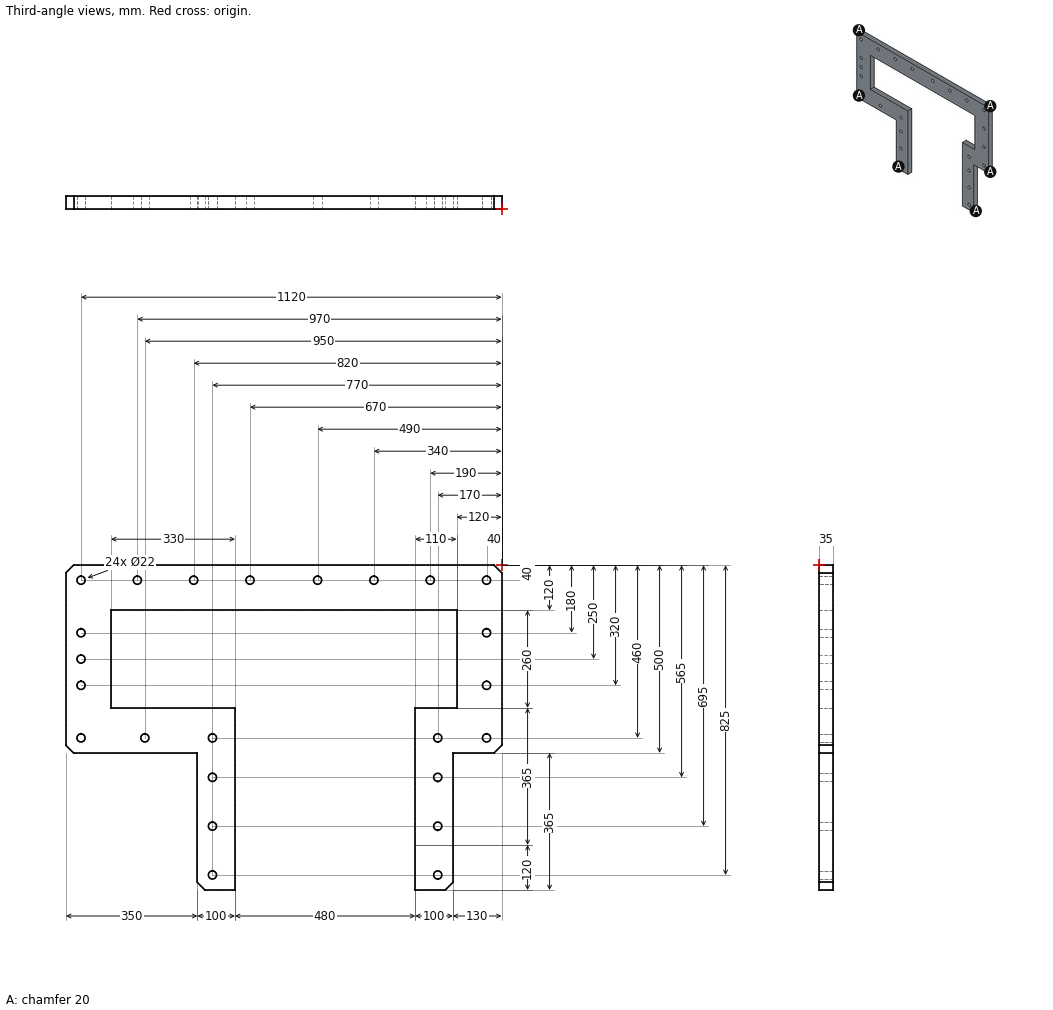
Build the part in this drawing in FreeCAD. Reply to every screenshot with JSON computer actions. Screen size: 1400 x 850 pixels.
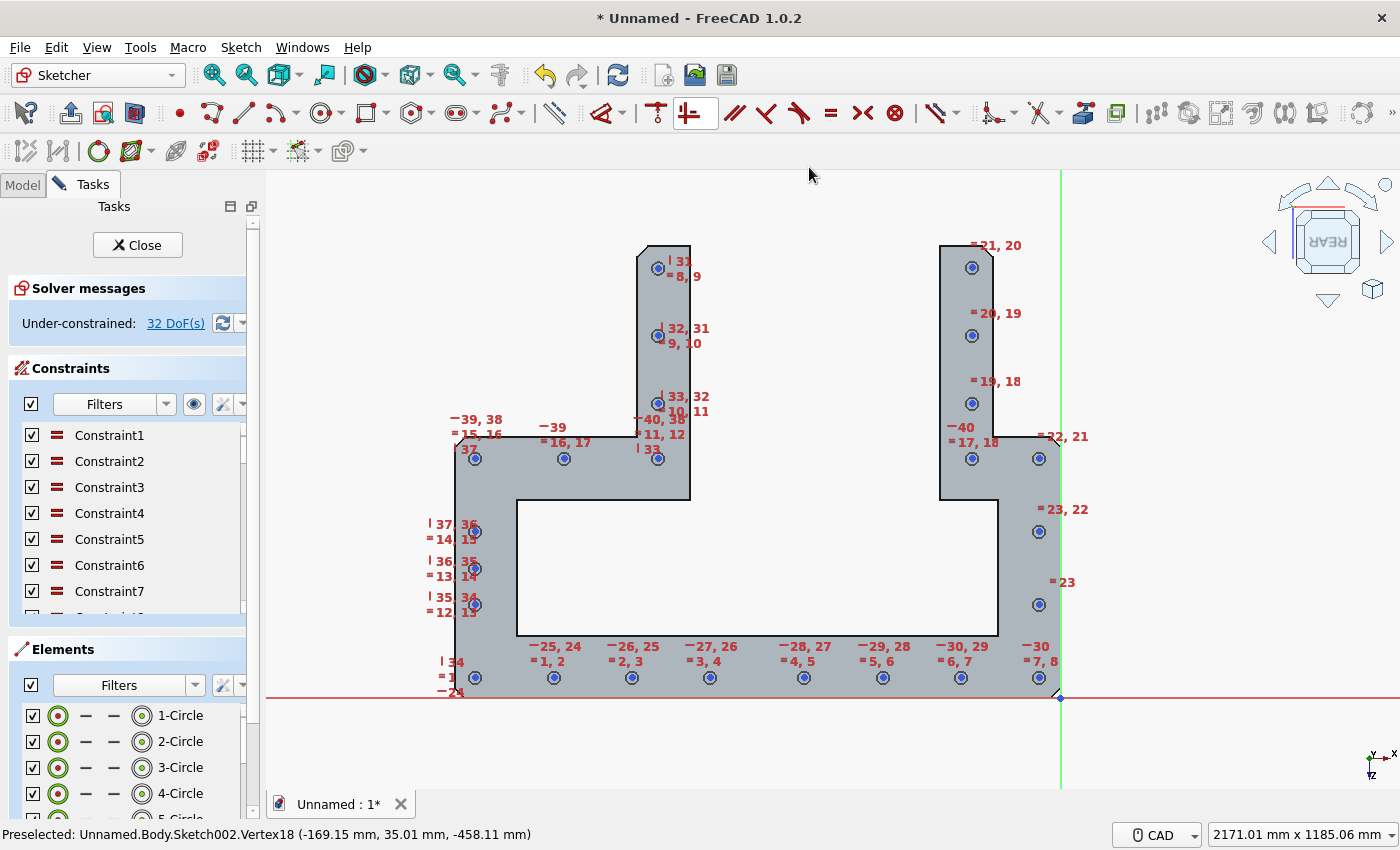
{"action": "left_click", "coordinate": [972, 459]}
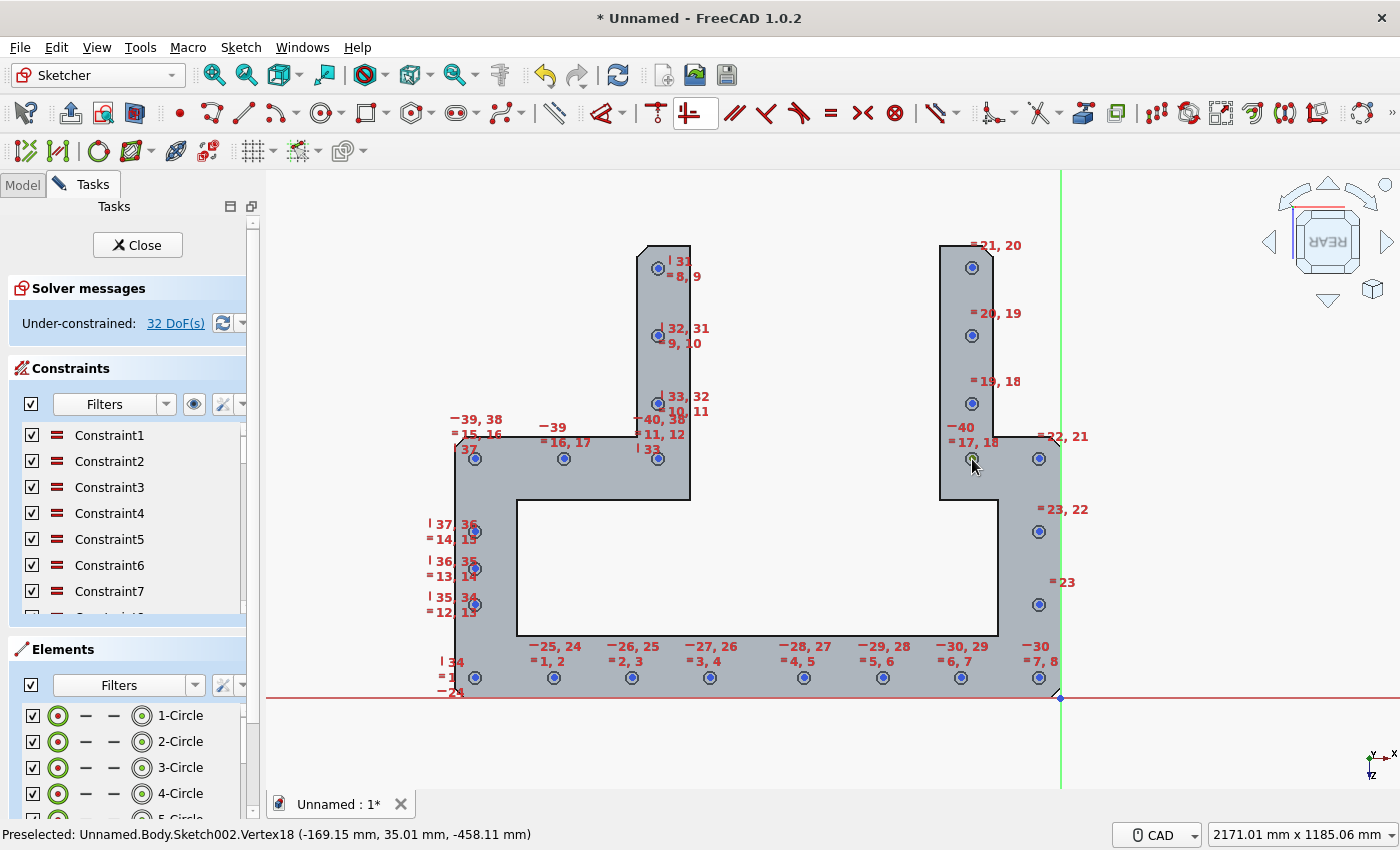
{"action": "left_click", "coordinate": [972, 404]}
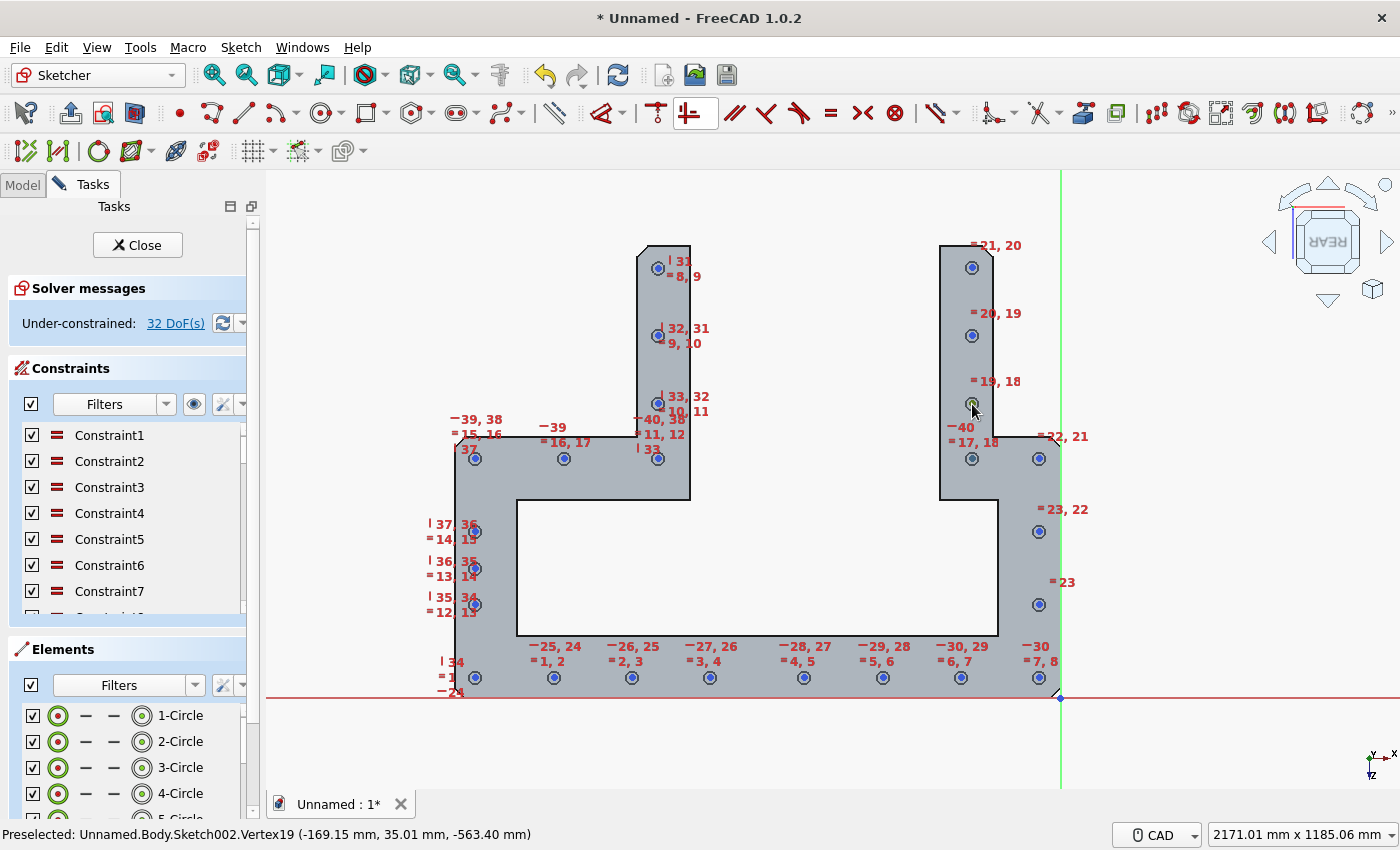
{"action": "key", "text": "v"}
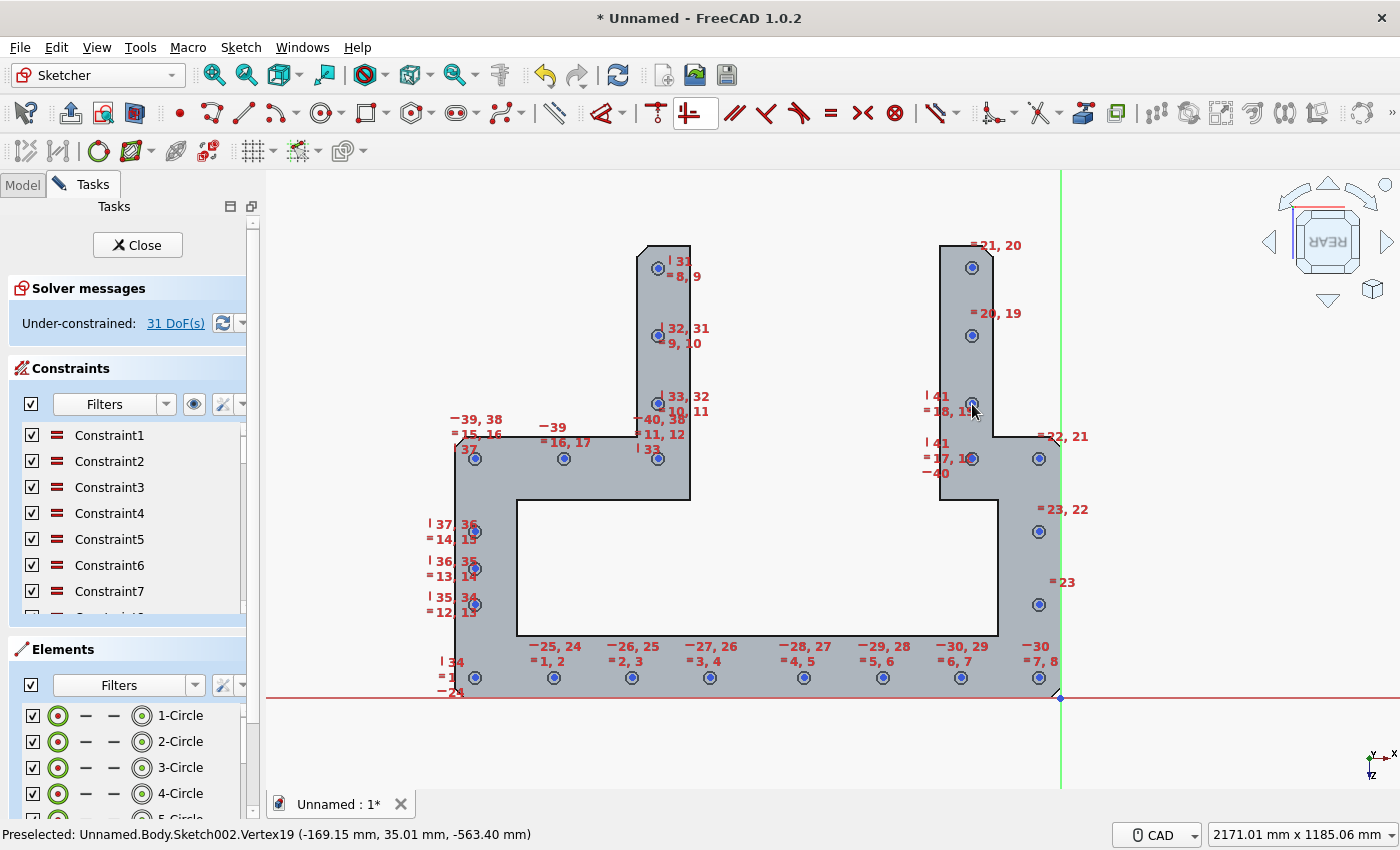
{"action": "left_click", "coordinate": [658, 404]}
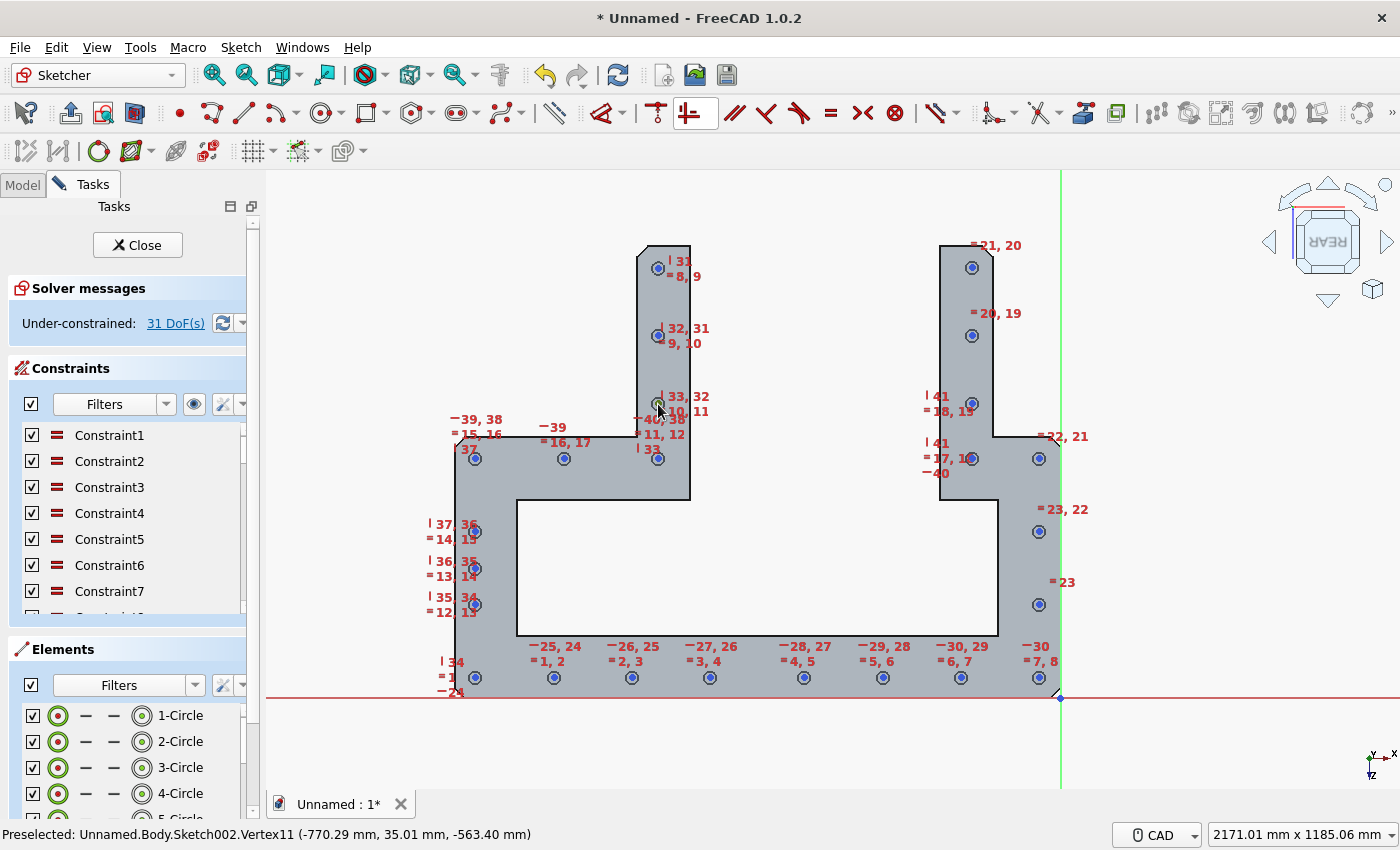
{"action": "left_click", "coordinate": [974, 406]}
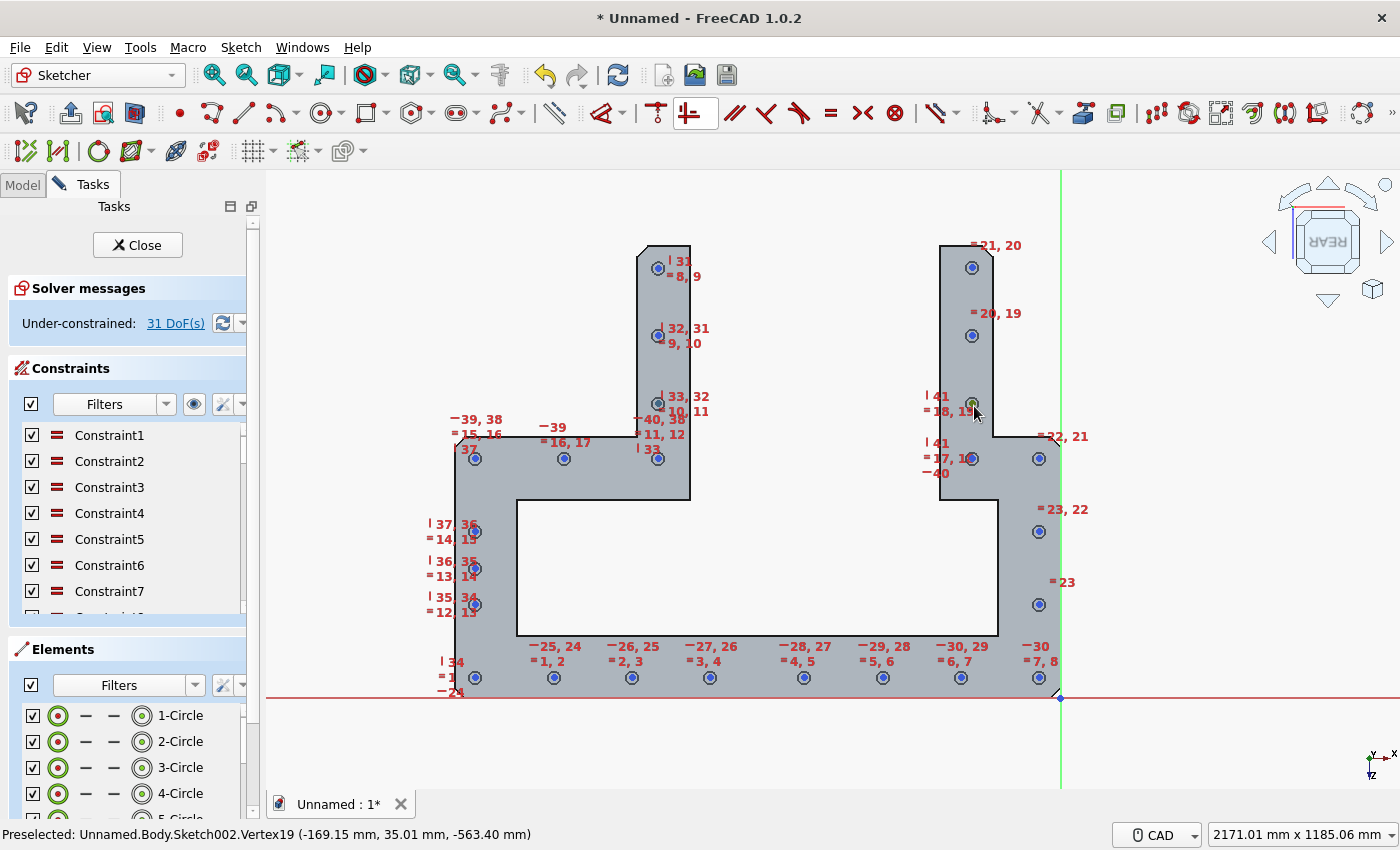
{"action": "key", "text": "h"}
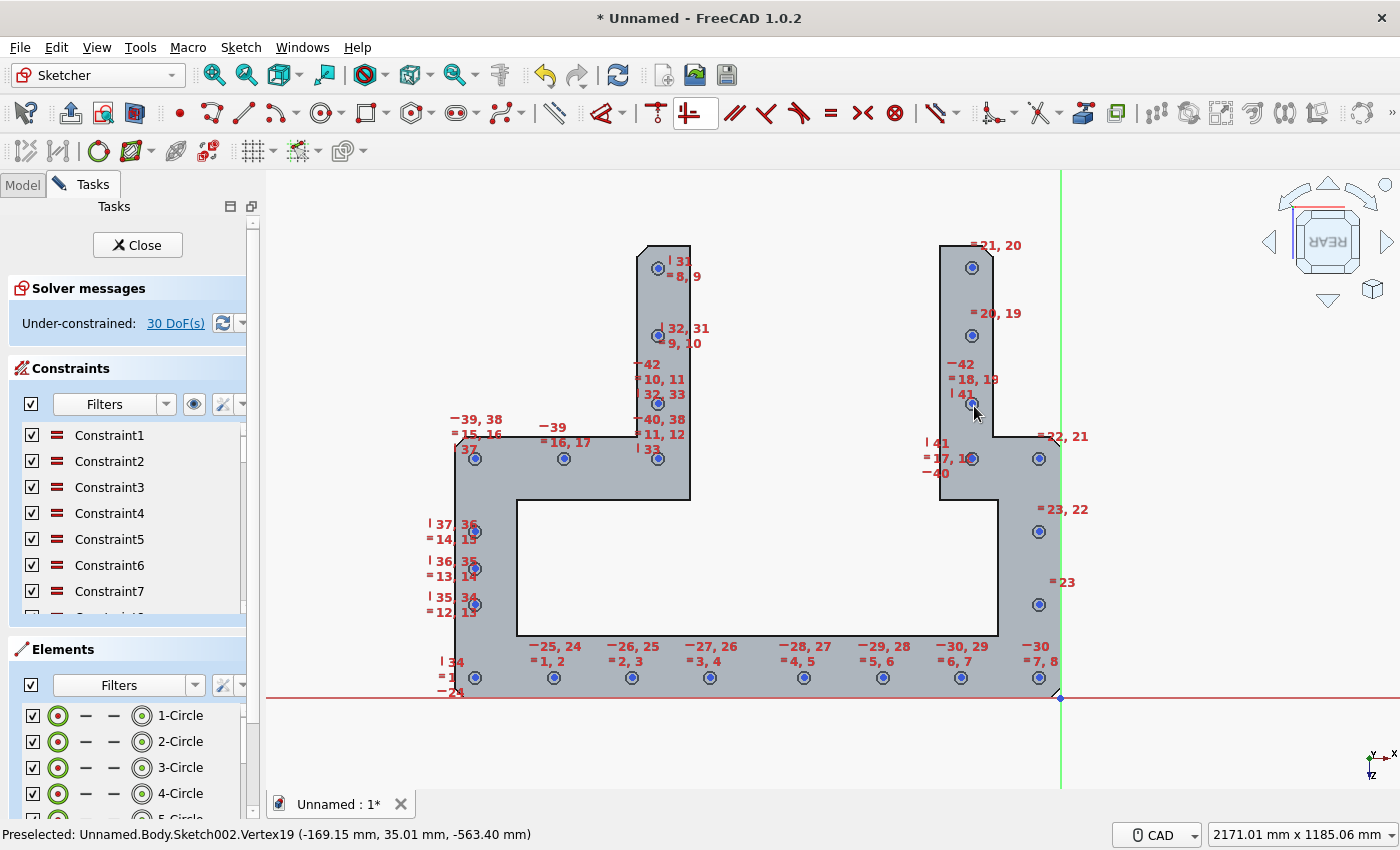
{"action": "left_click", "coordinate": [972, 404]}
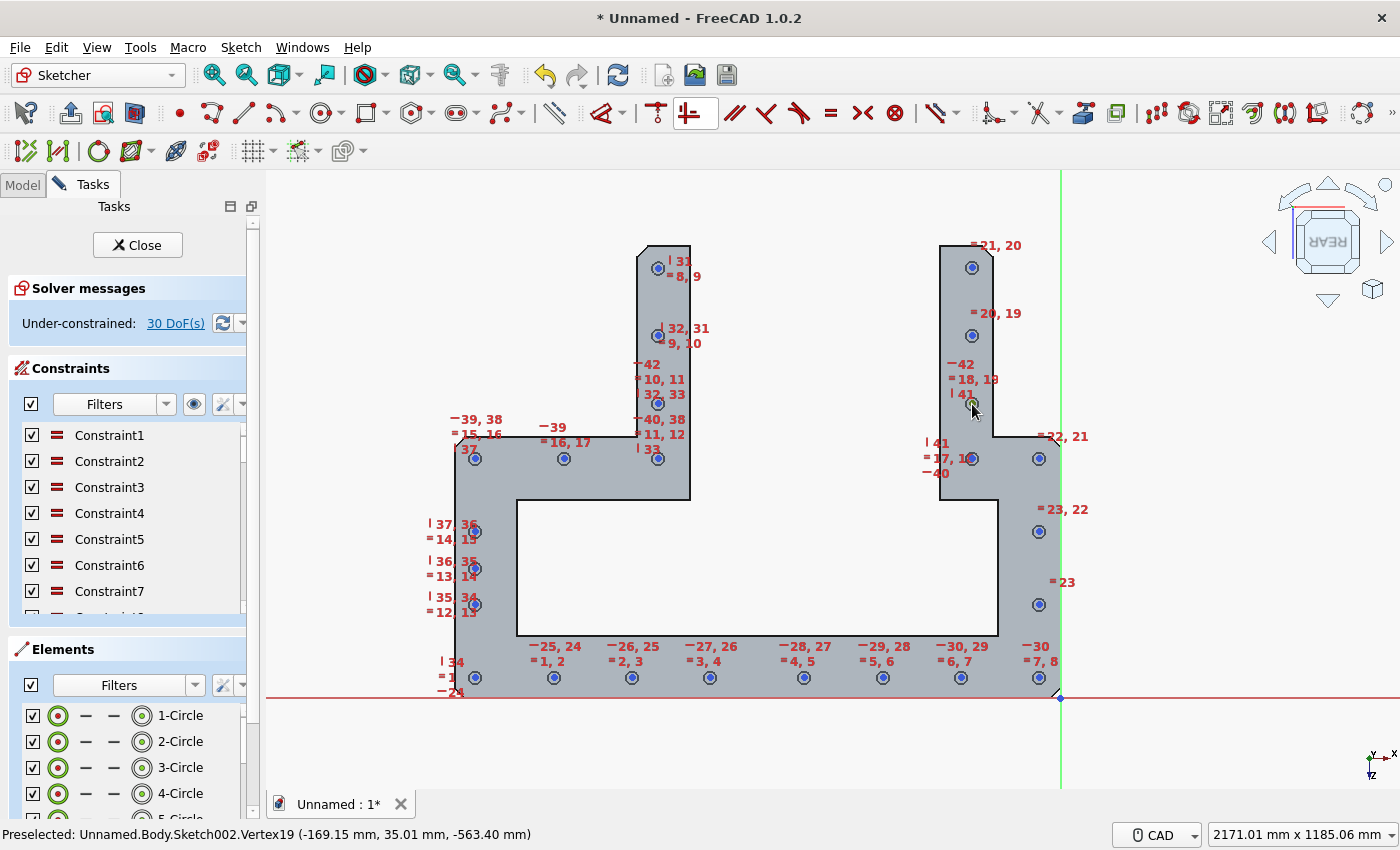
{"action": "left_click", "coordinate": [972, 336]}